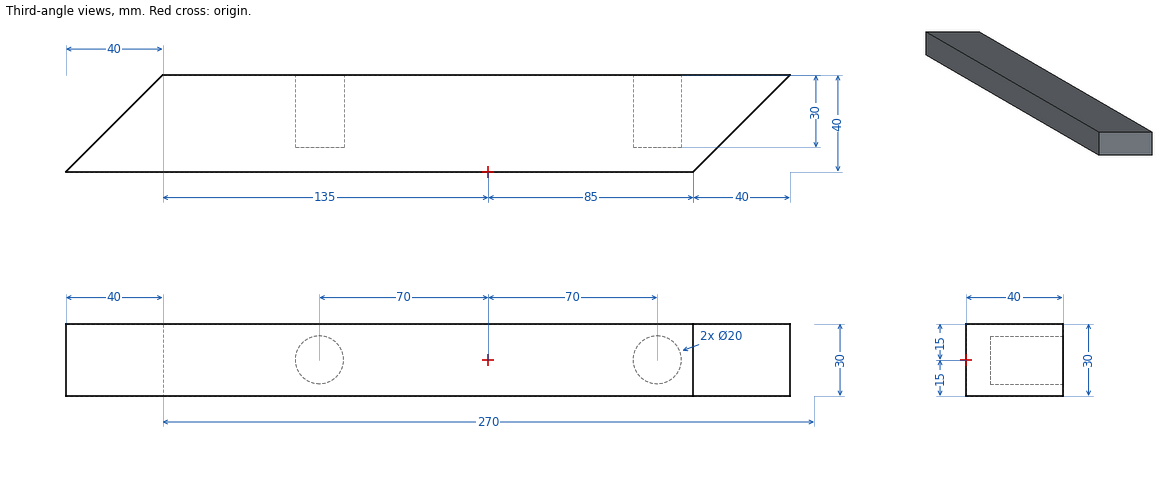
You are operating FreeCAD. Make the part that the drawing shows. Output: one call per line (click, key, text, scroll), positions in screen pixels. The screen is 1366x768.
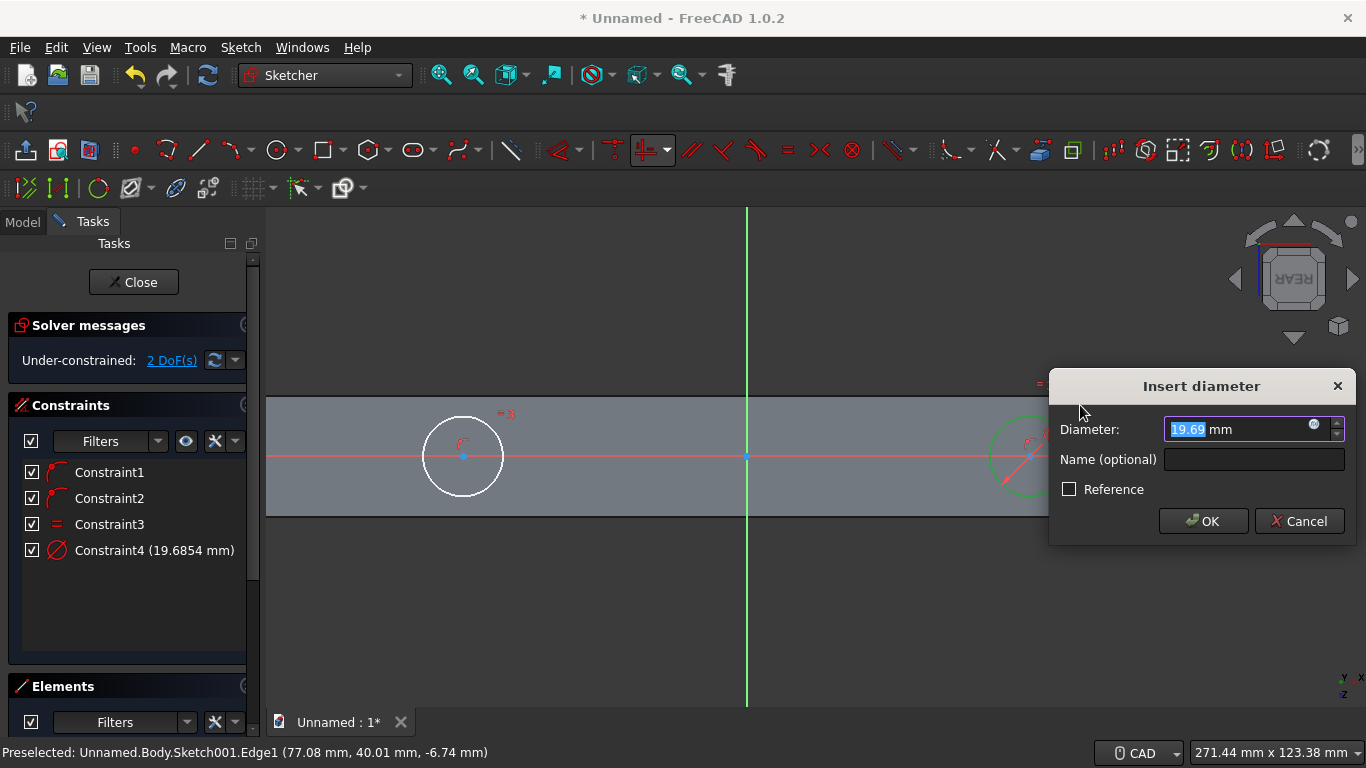
text(20)
key(Return)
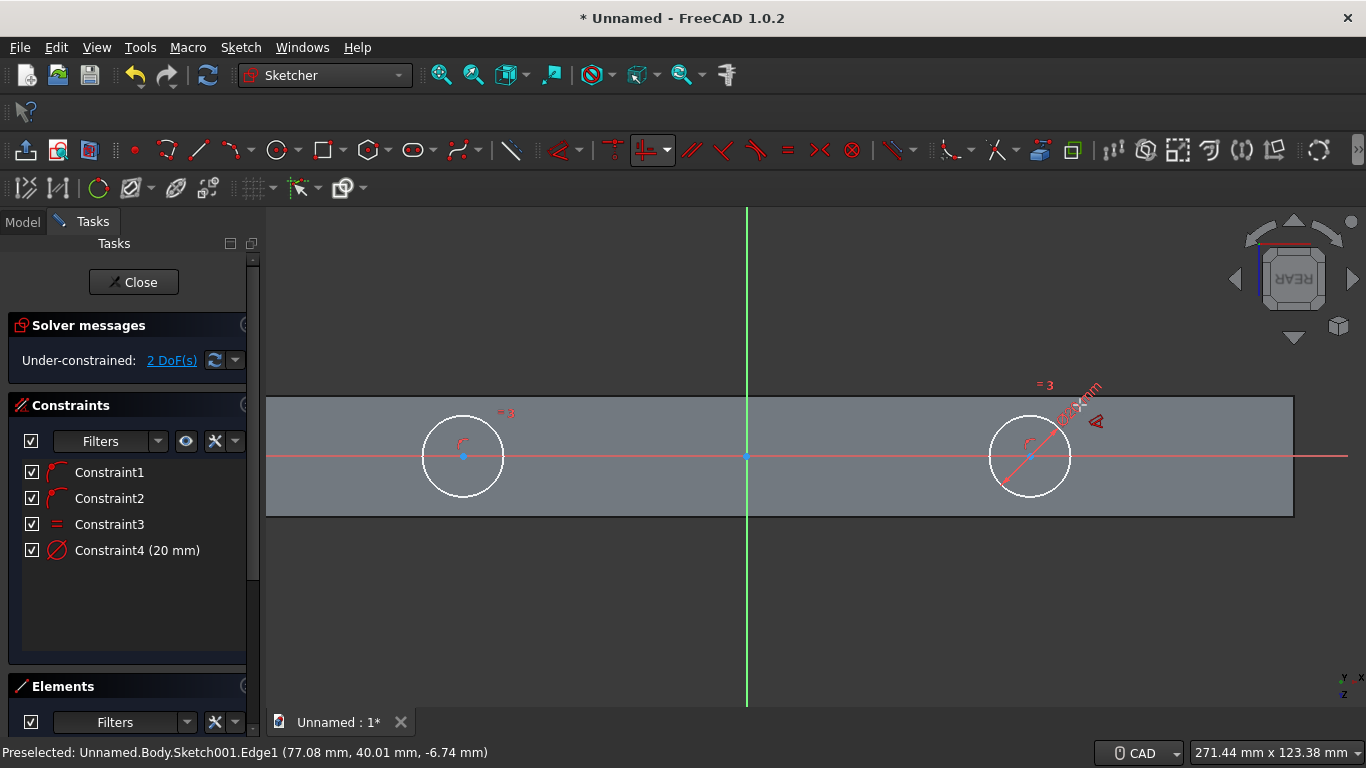
click(1030, 456)
click(888, 490)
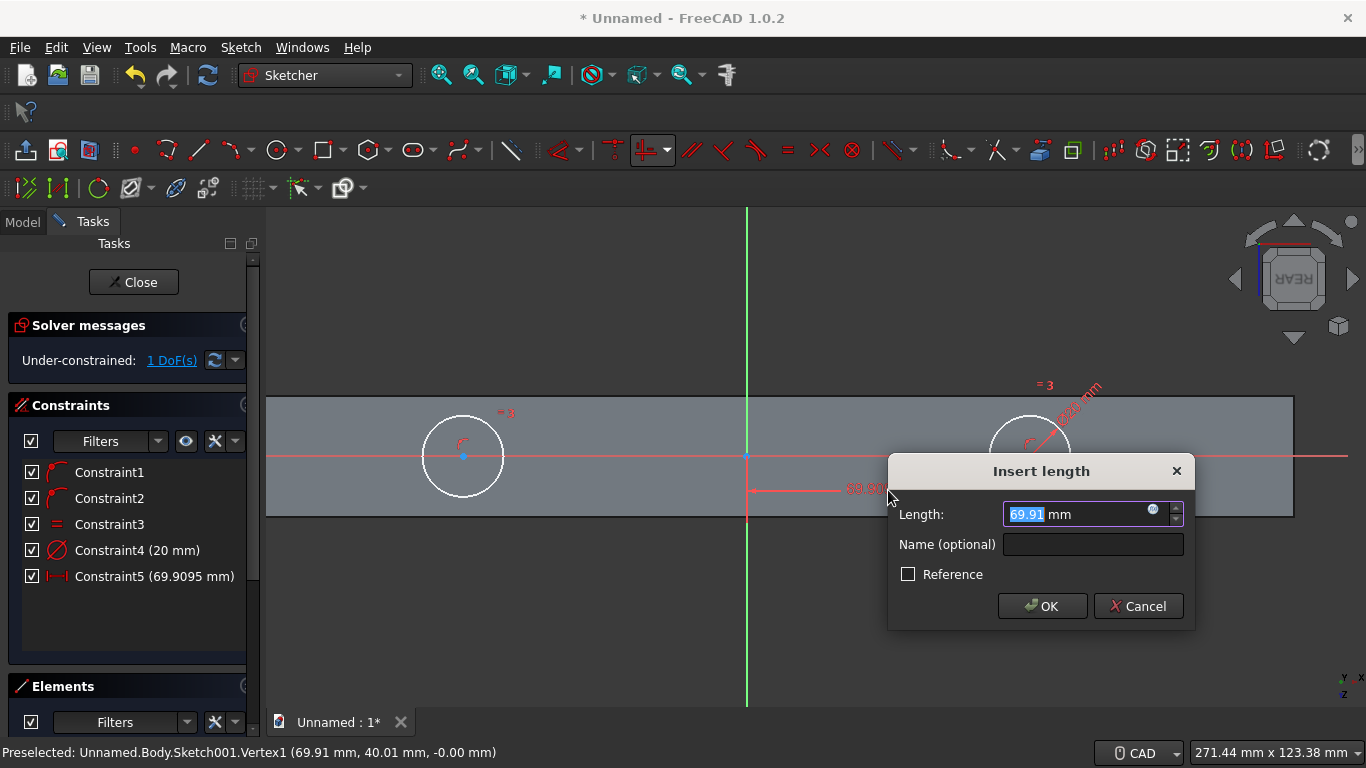
text(70)
key(Return)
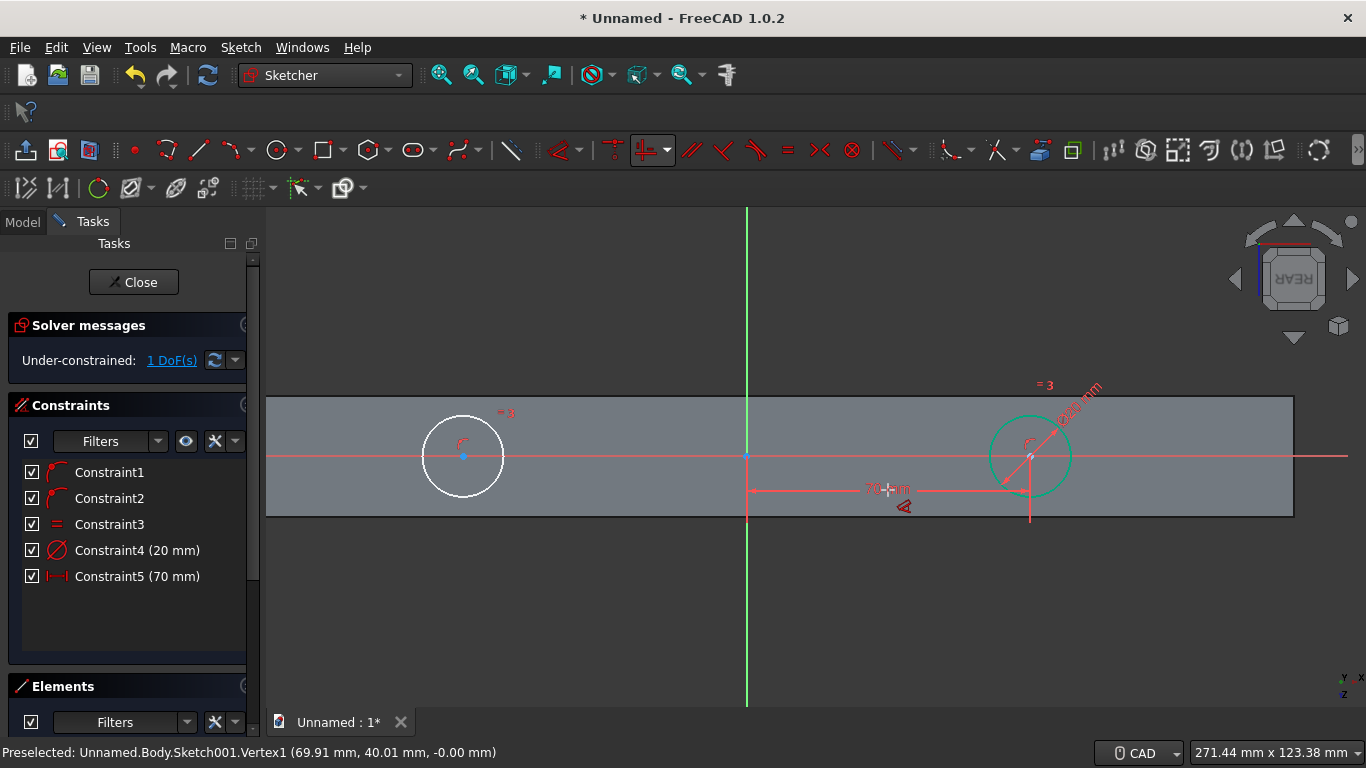
click(463, 456)
click(605, 490)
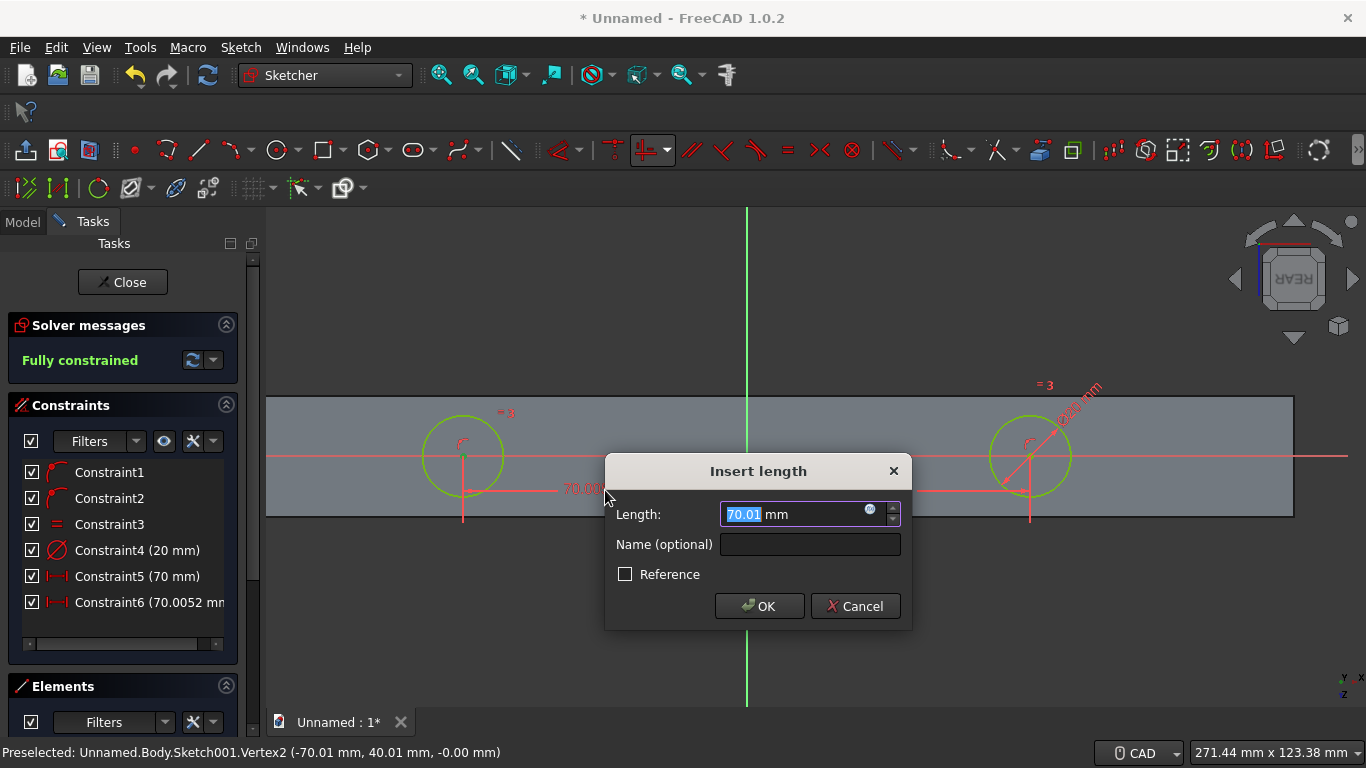
text(70)
key(Return)
key(Escape)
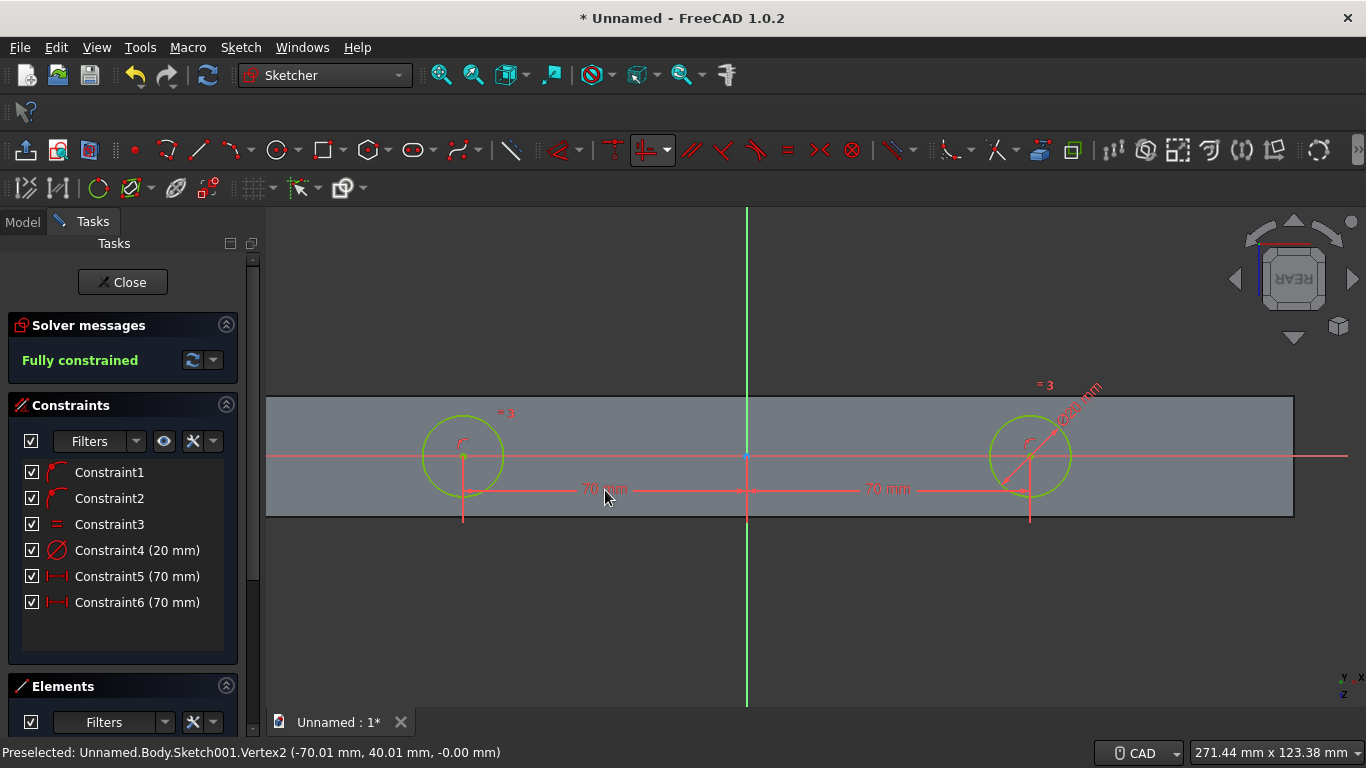
click(123, 282)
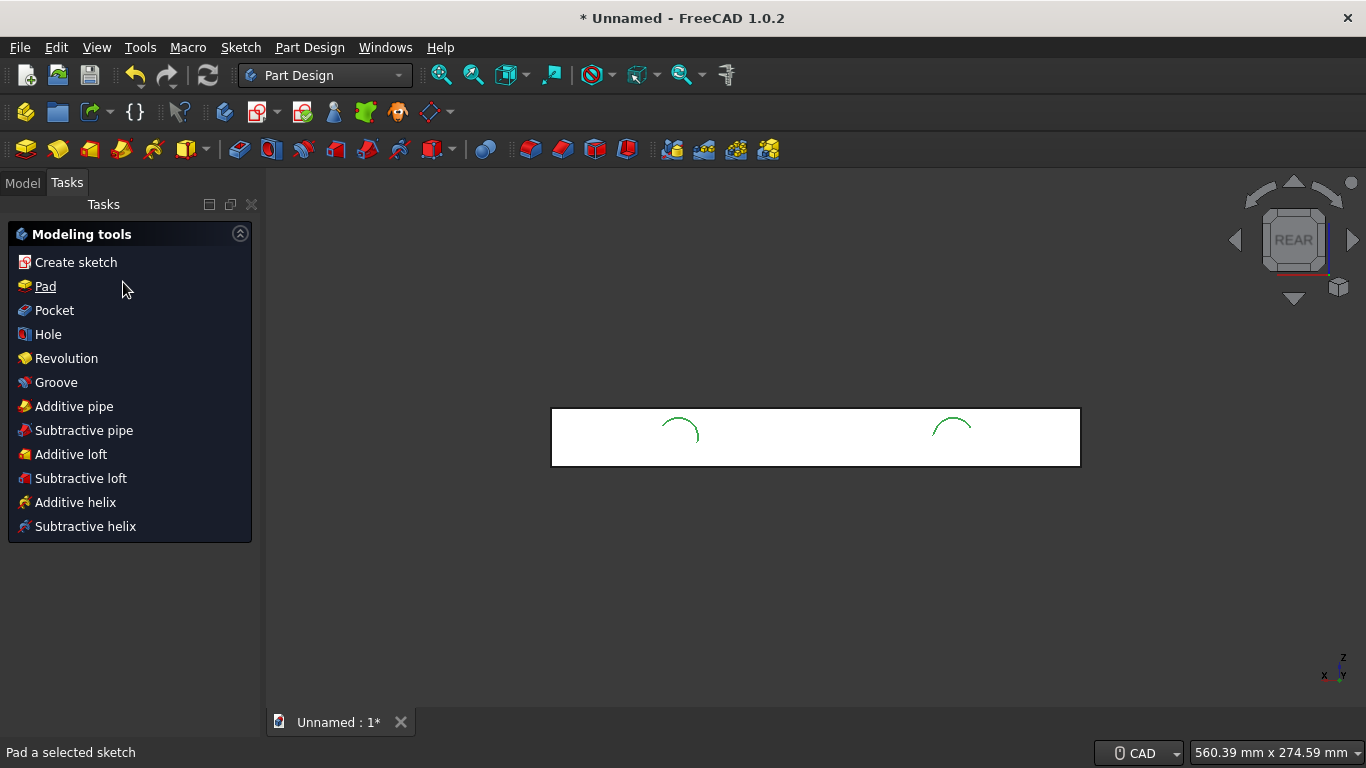
click(240, 150)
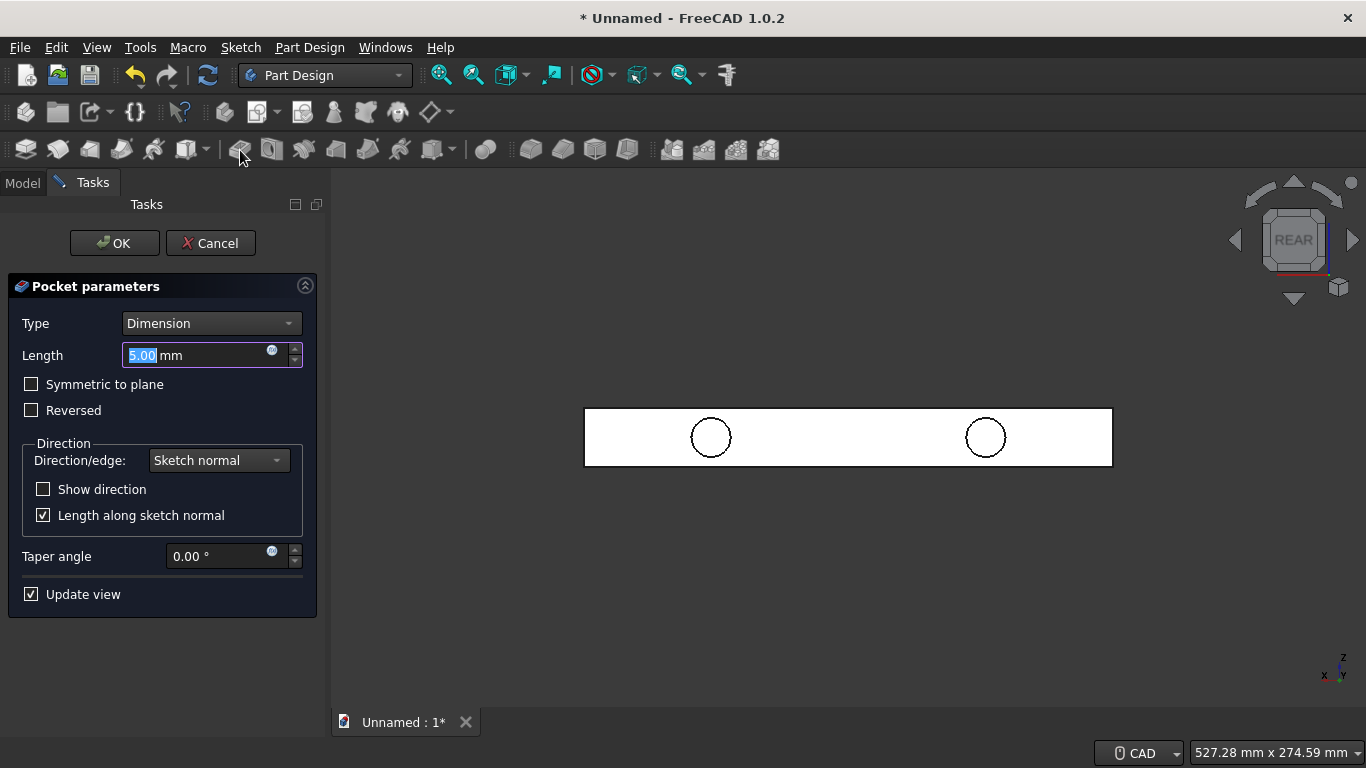
text(30)
key(Tab)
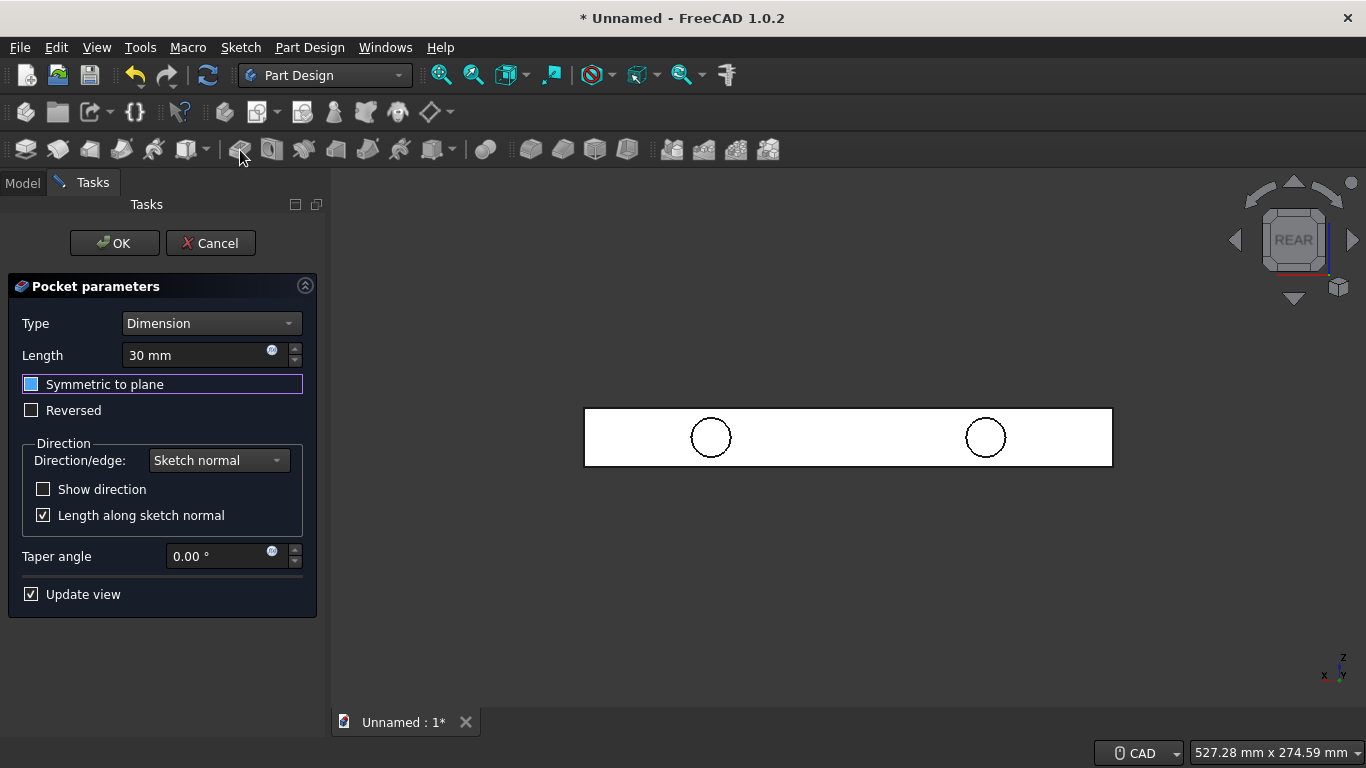
click(115, 243)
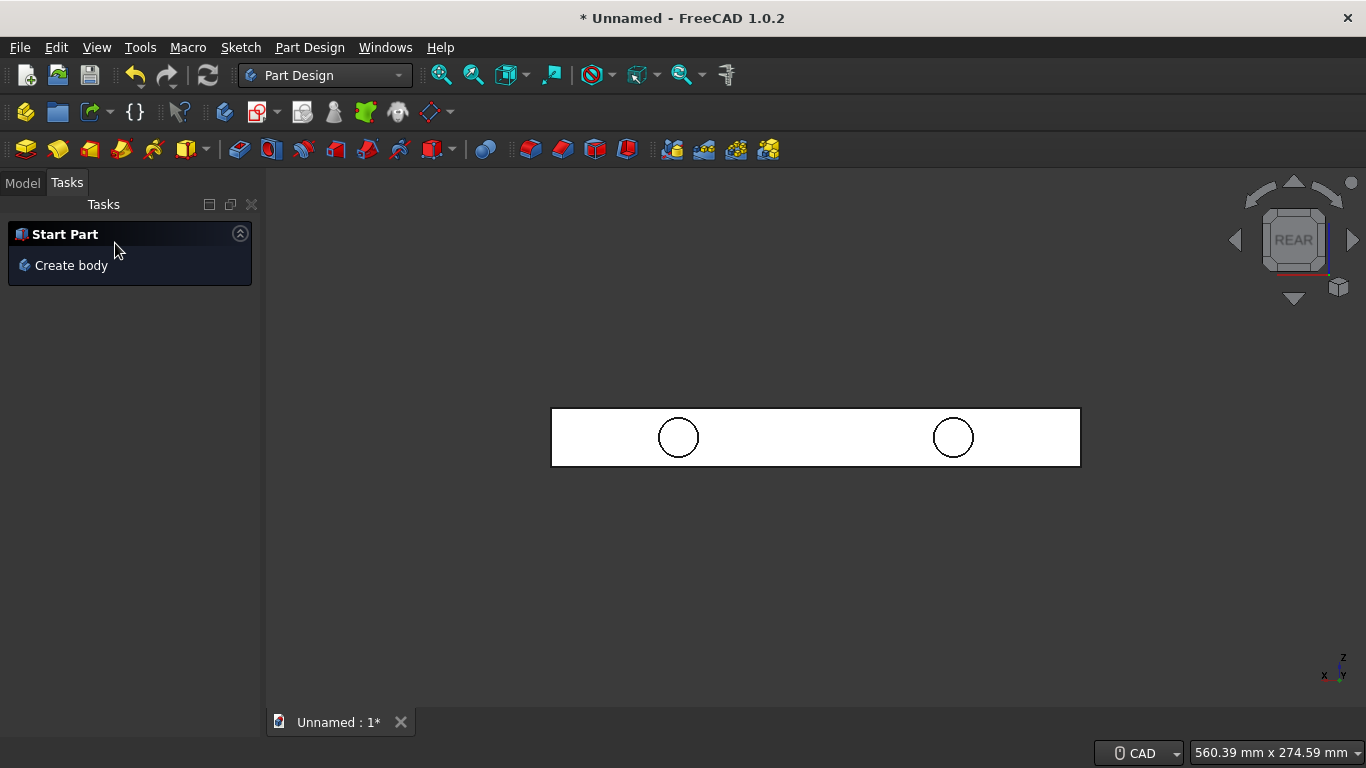
key(0)